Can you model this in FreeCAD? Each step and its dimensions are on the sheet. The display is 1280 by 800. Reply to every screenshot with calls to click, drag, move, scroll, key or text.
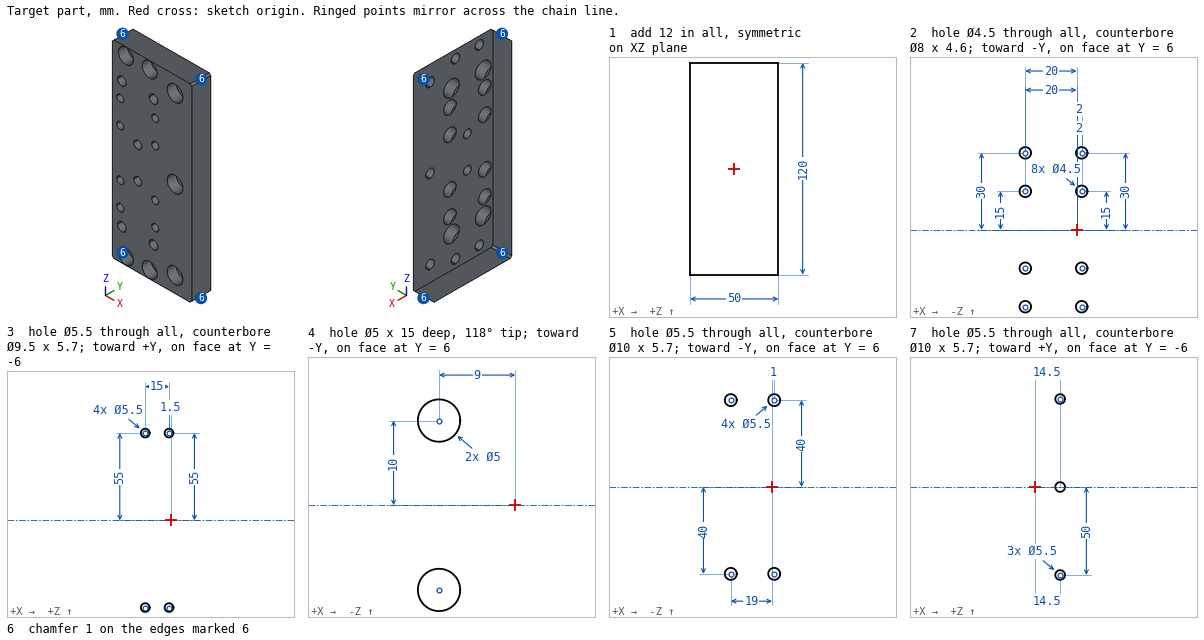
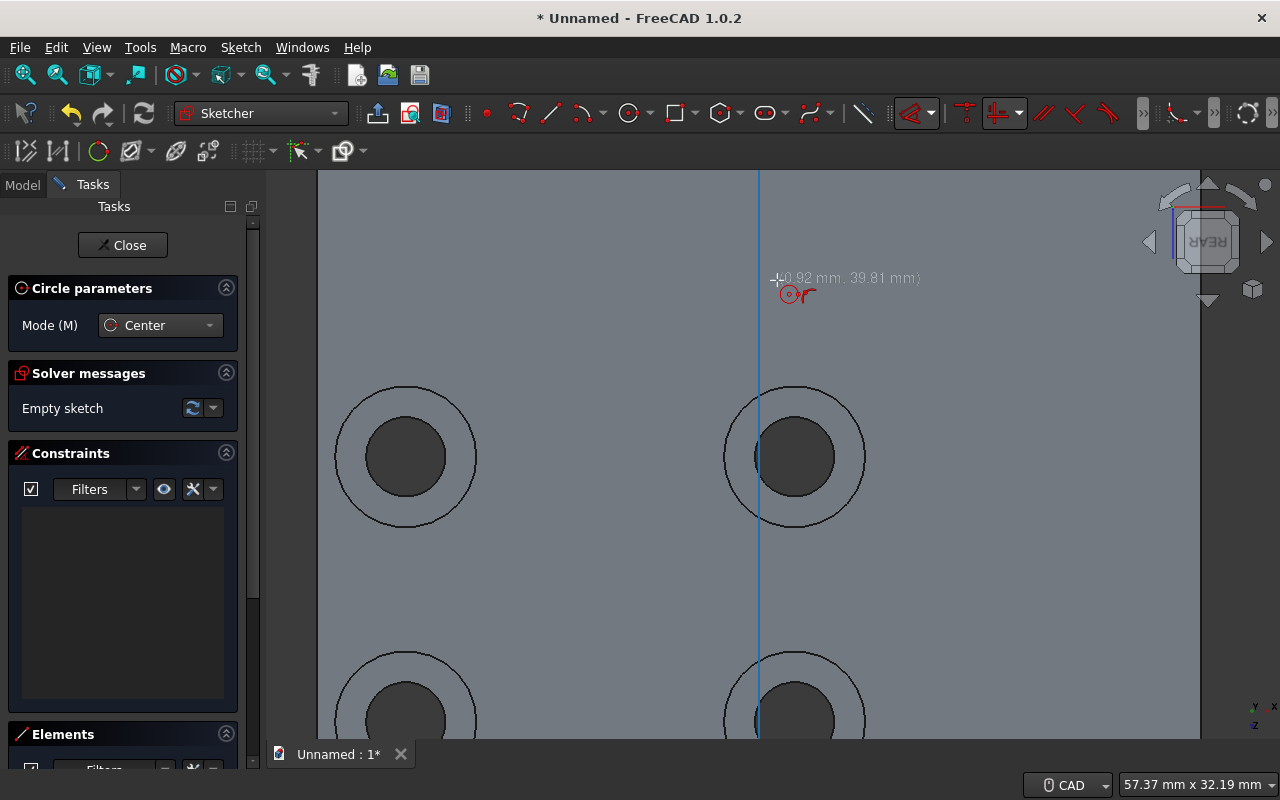
click(777, 280)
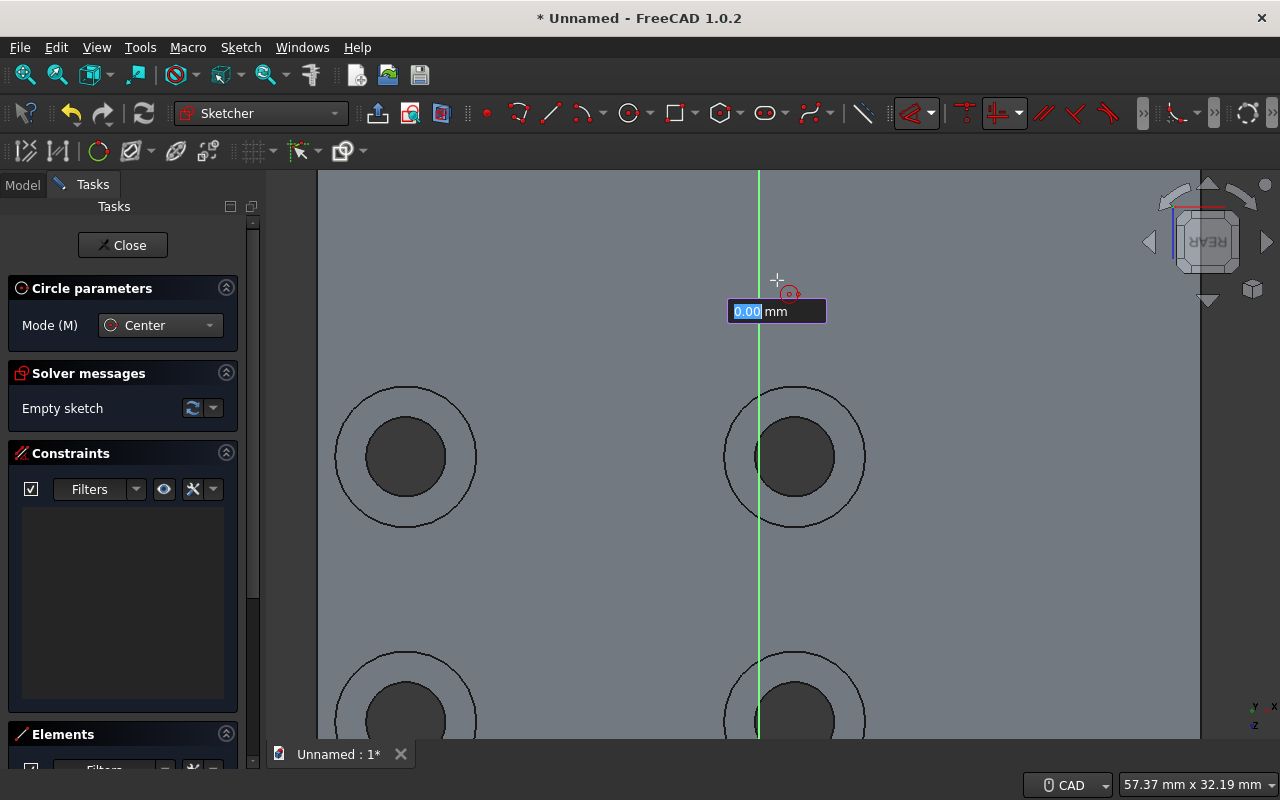
scroll(739, 280, down, 7)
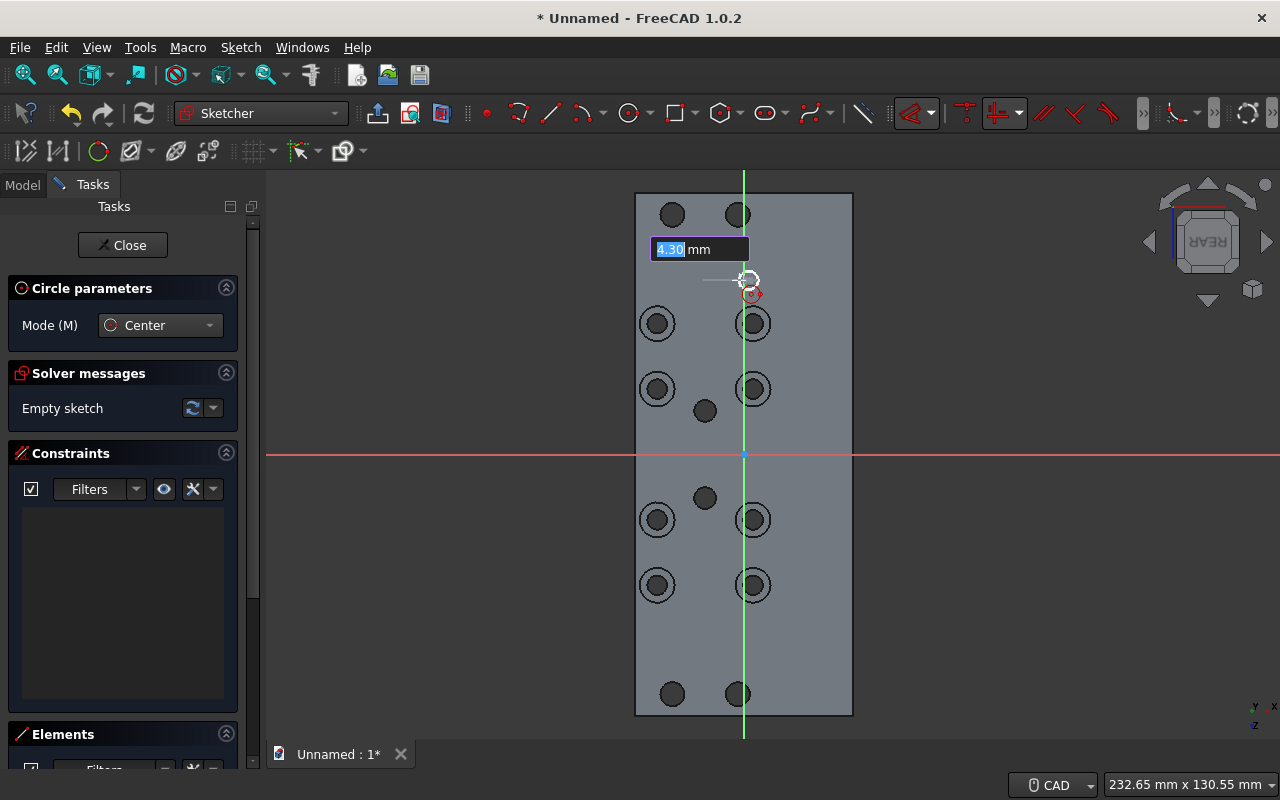
scroll(757, 272, up, 2)
move(757, 271)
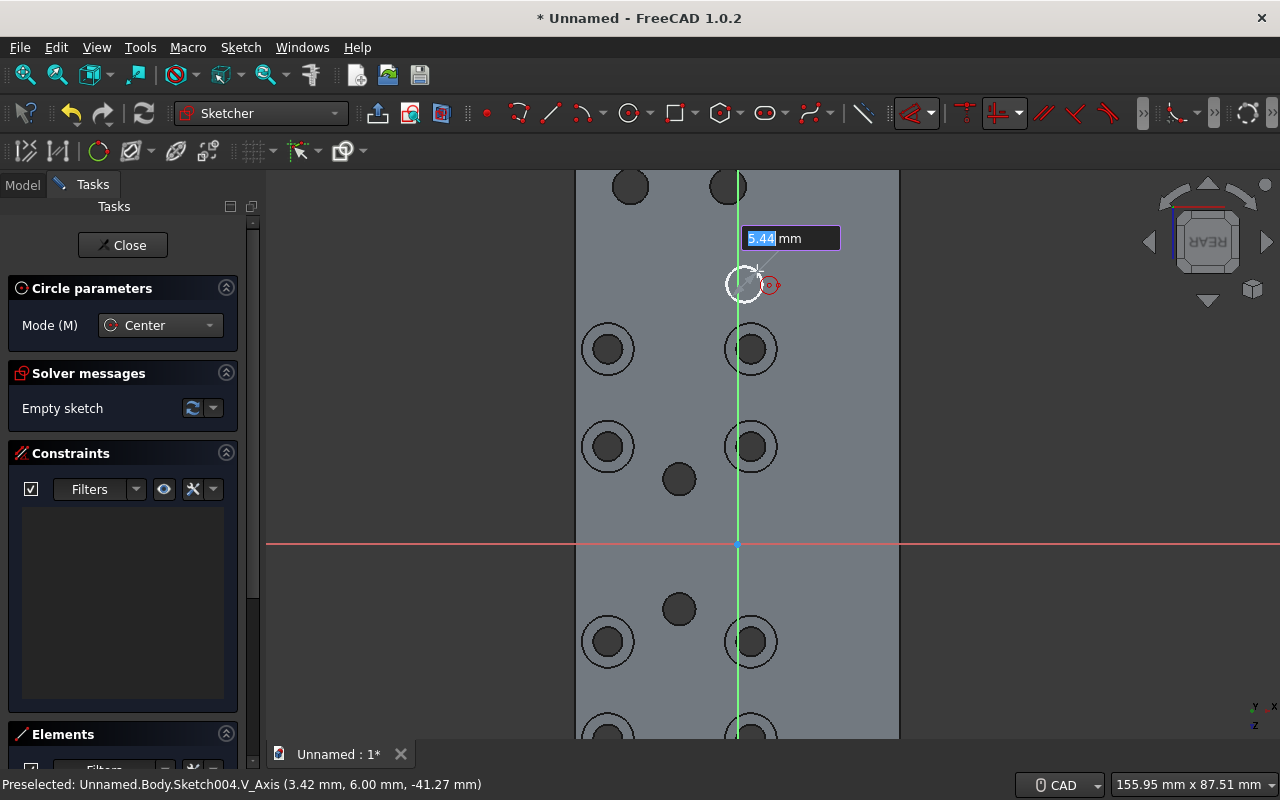
text(5.5)
key(Return)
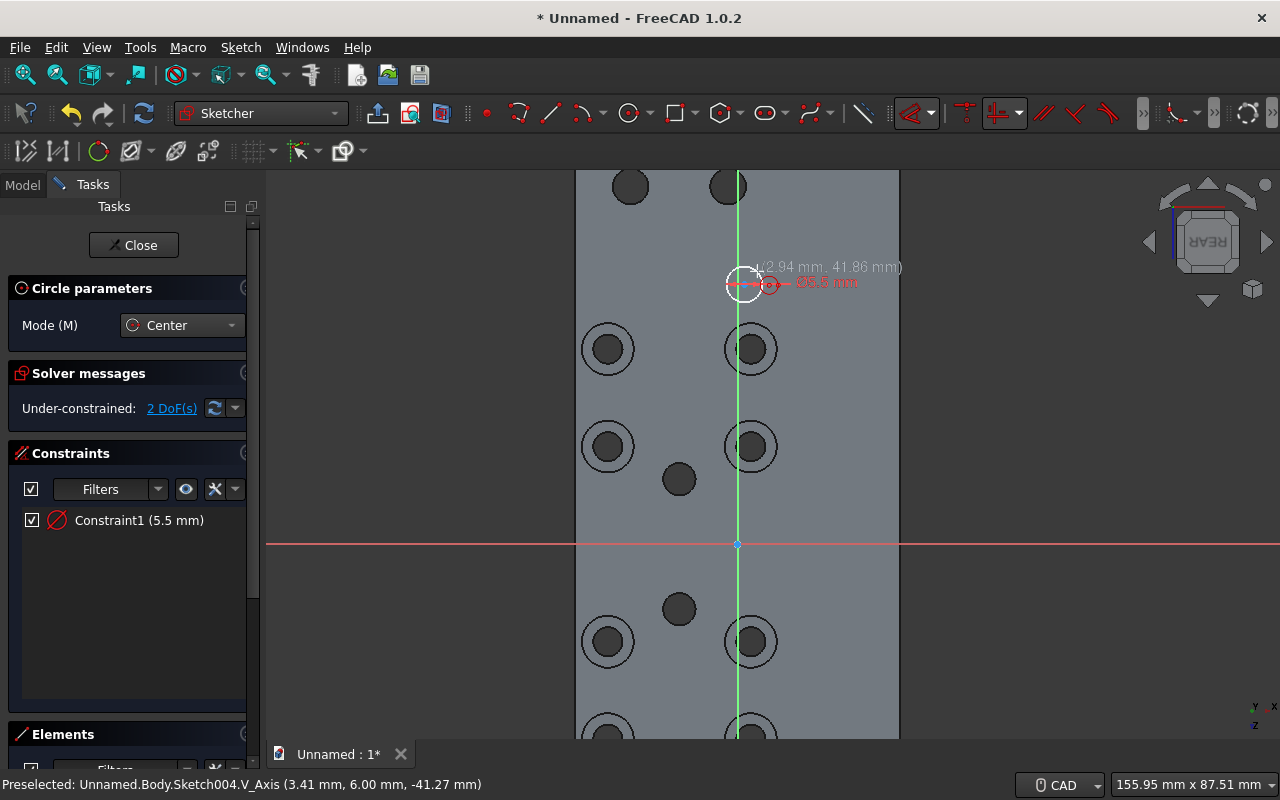
scroll(756, 272, down, 2)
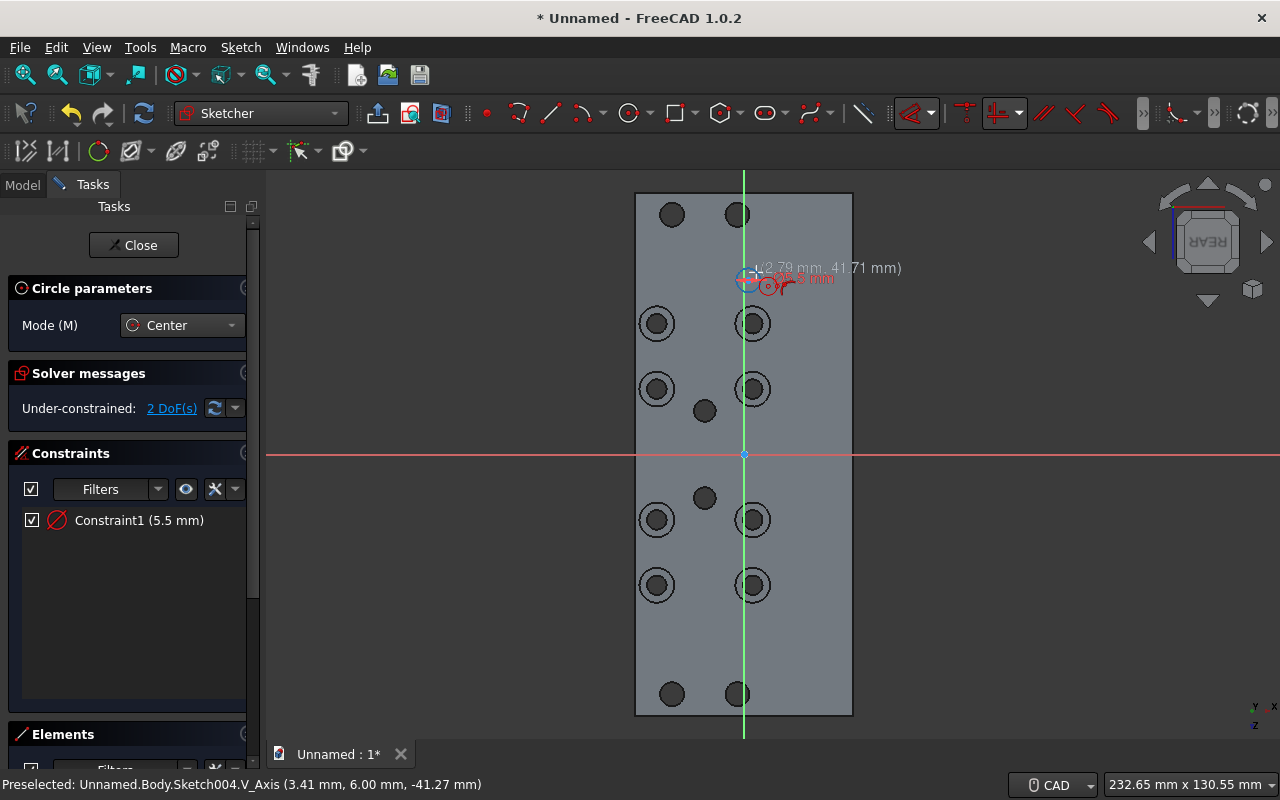
scroll(748, 629, up, 7)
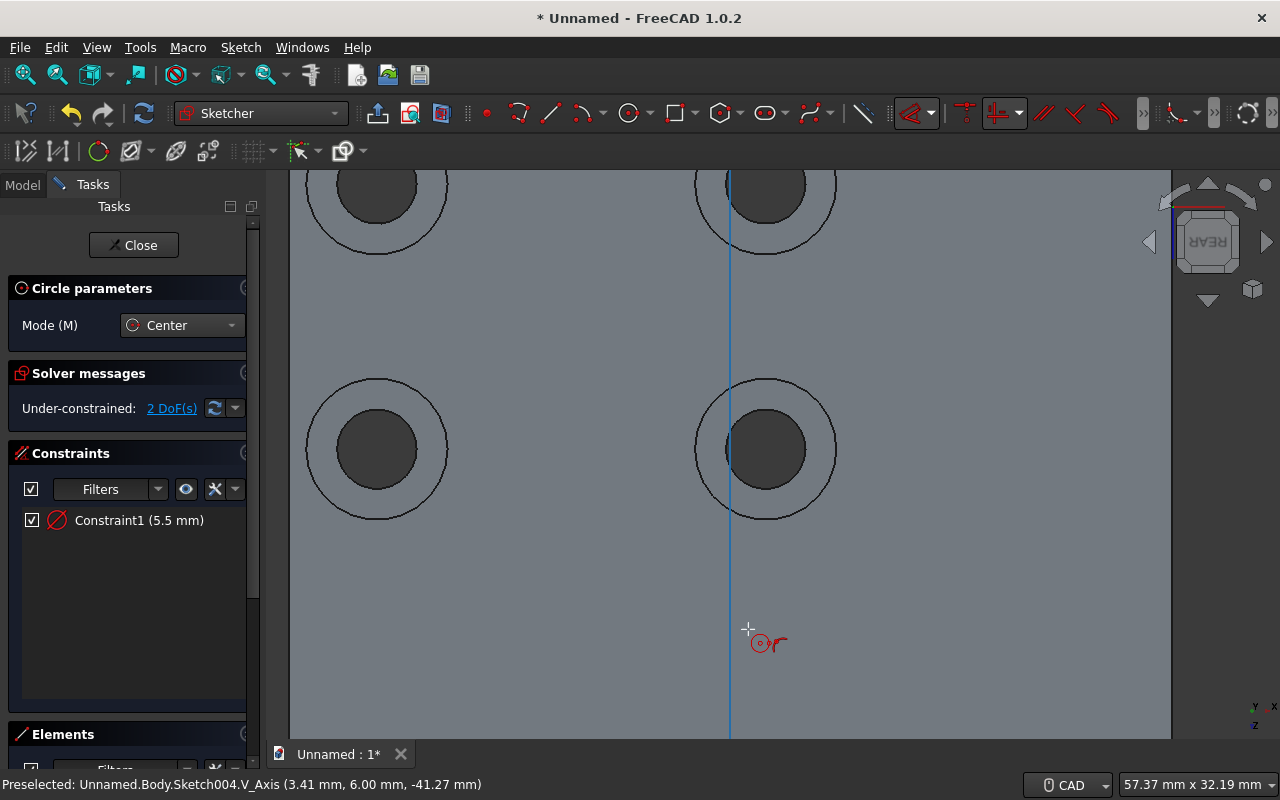
click(748, 626)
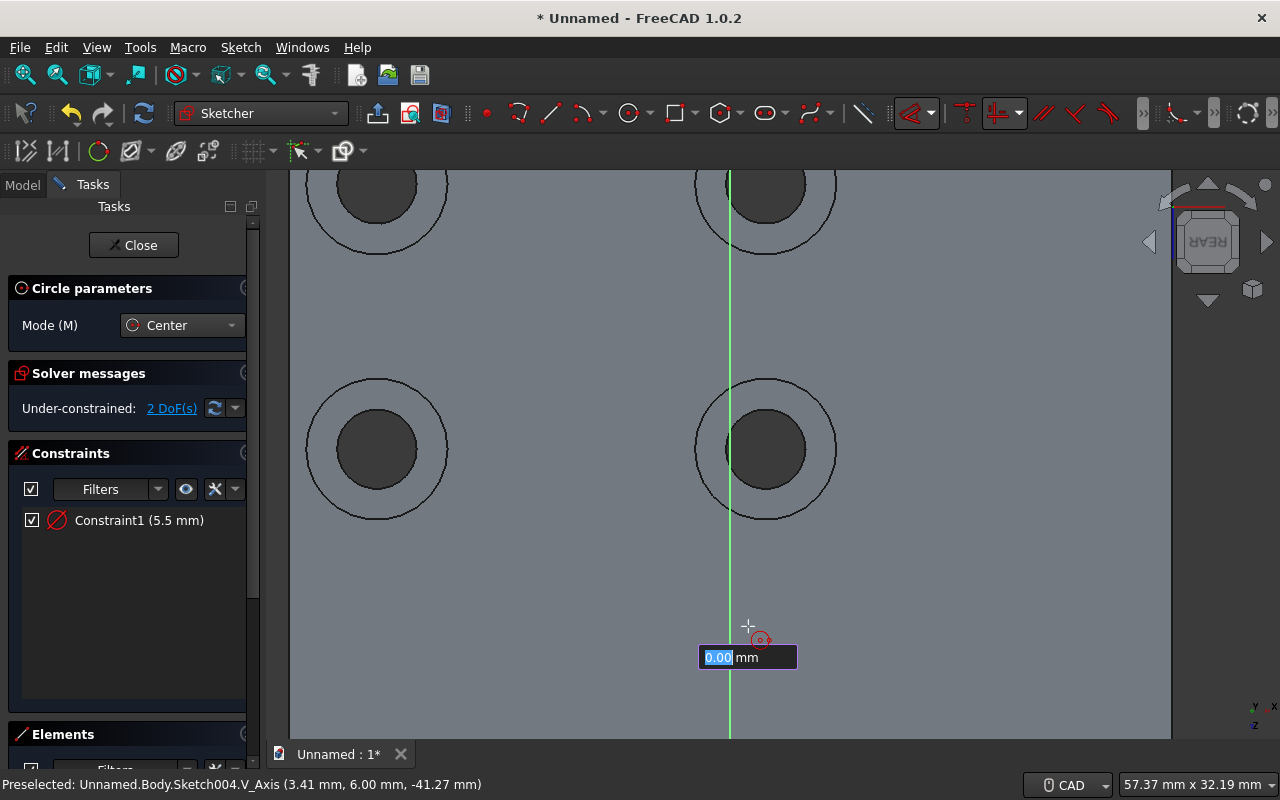
scroll(748, 630, down, 7)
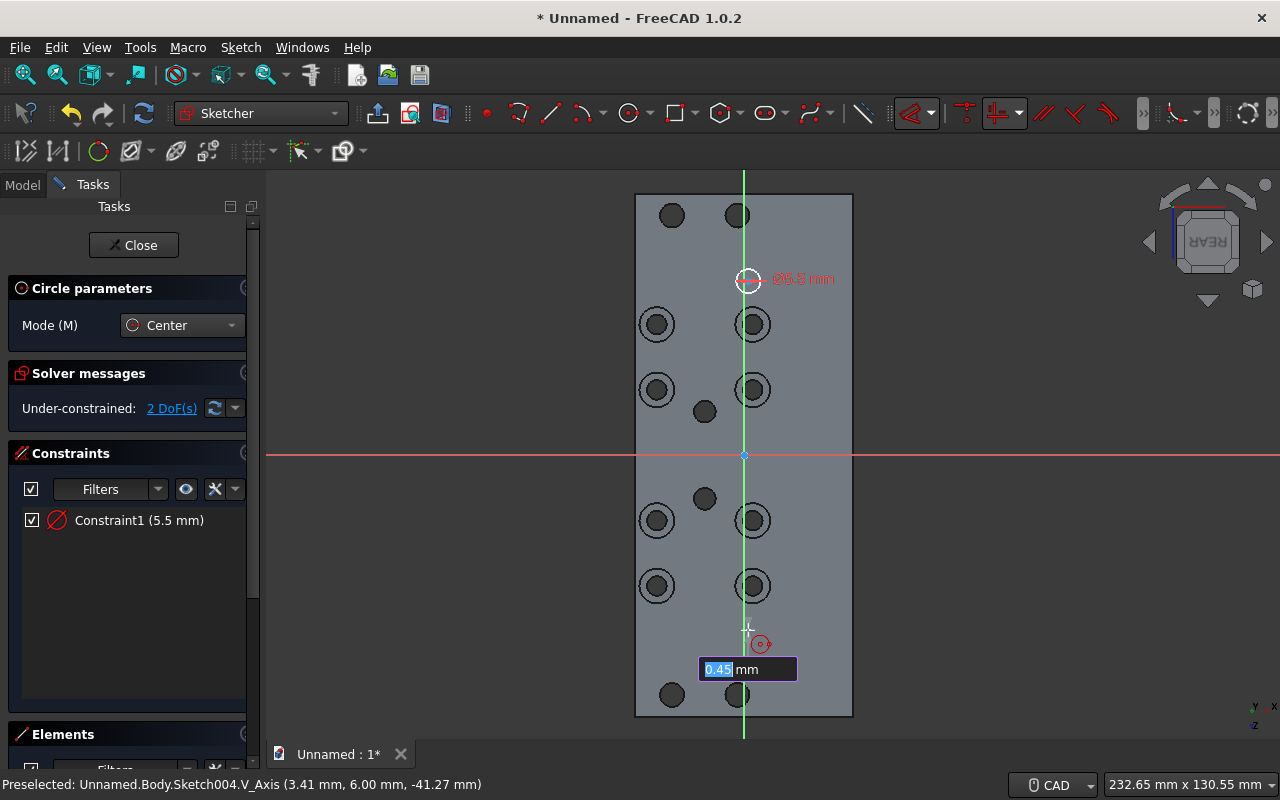
scroll(757, 621, up, 2)
move(757, 621)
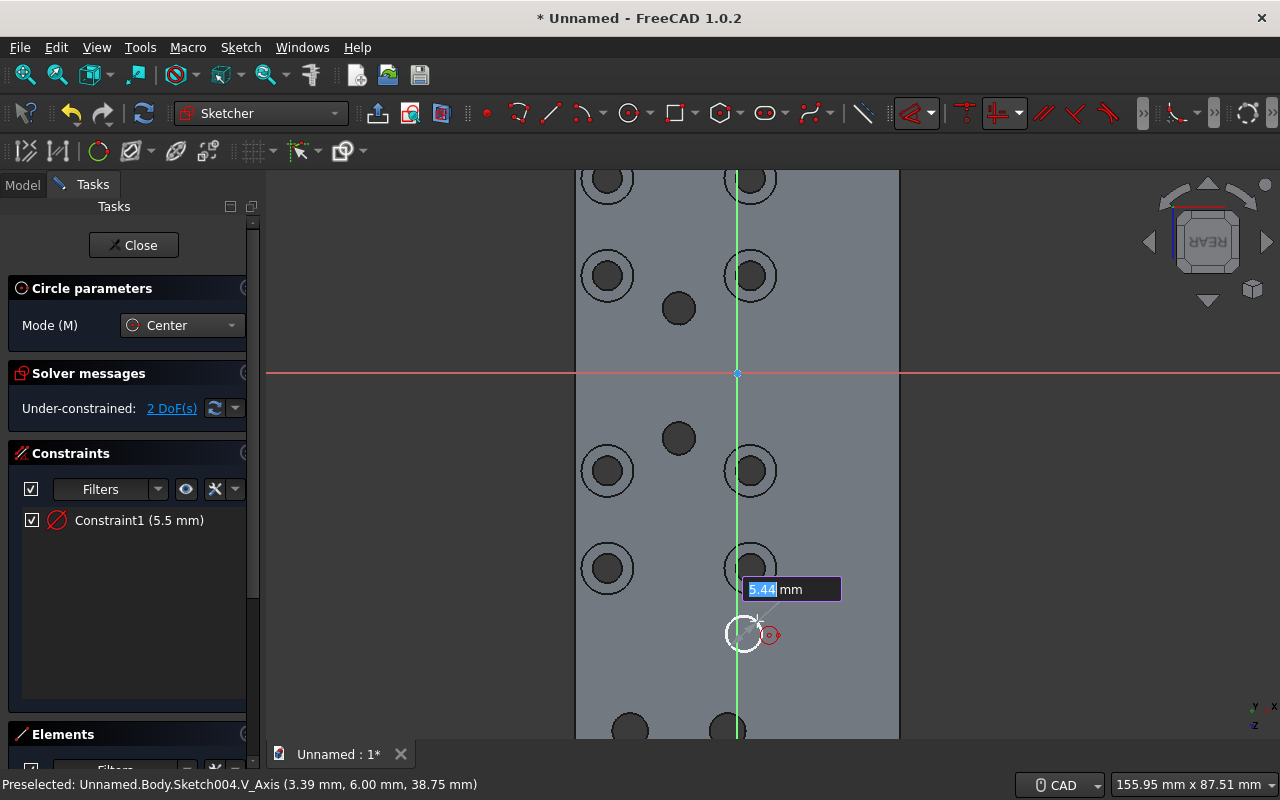
text(5.5)
key(Return)